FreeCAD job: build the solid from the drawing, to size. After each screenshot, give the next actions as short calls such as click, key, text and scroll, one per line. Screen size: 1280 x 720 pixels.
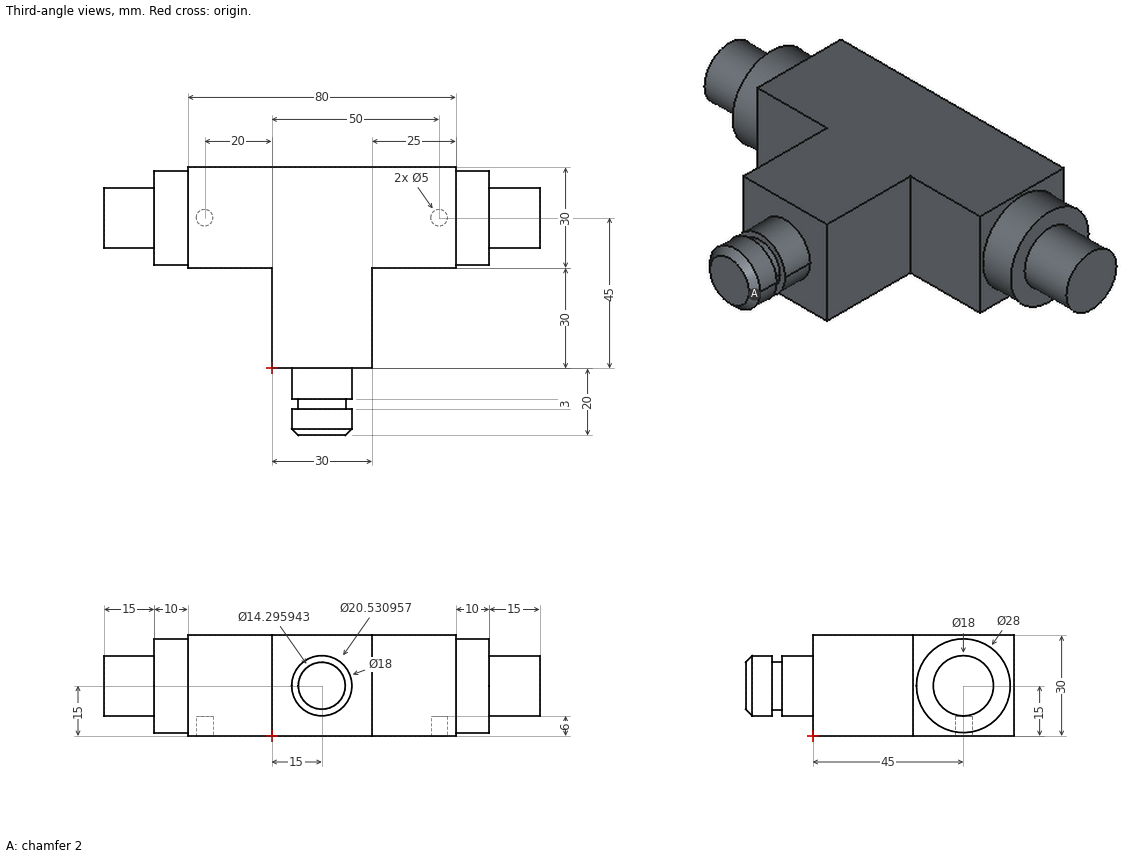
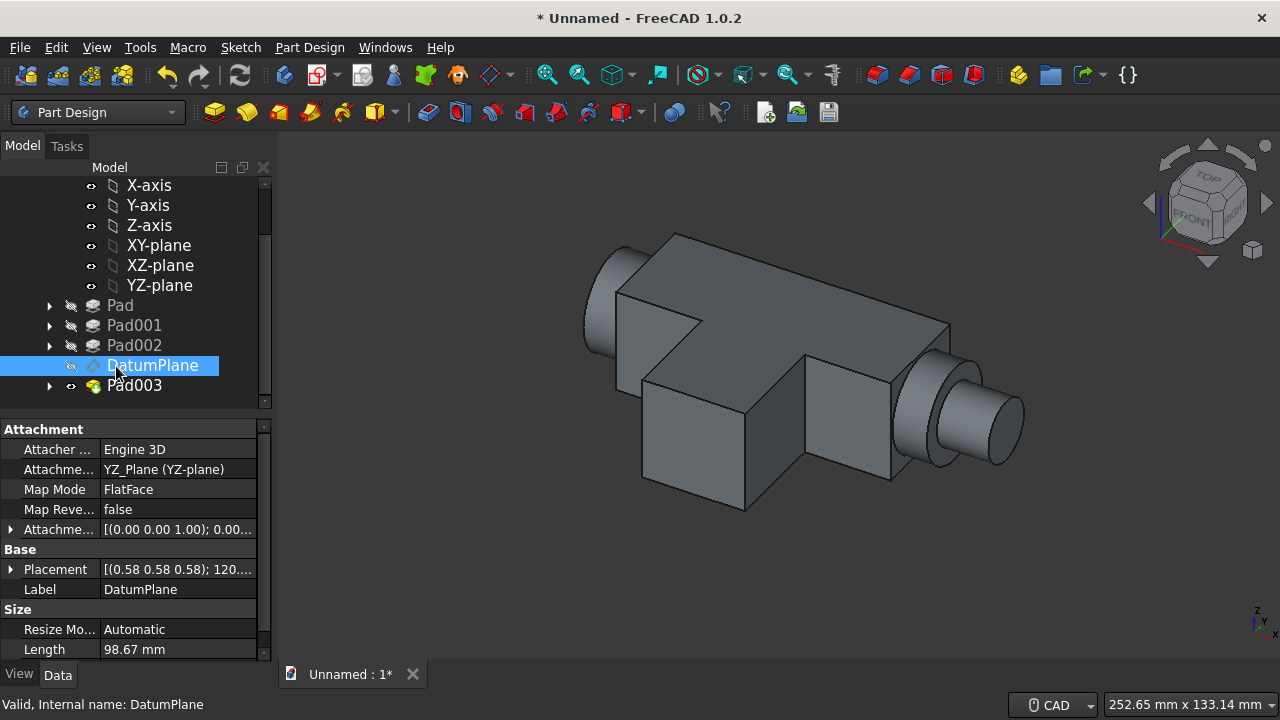
scroll(160, 281, down, 3)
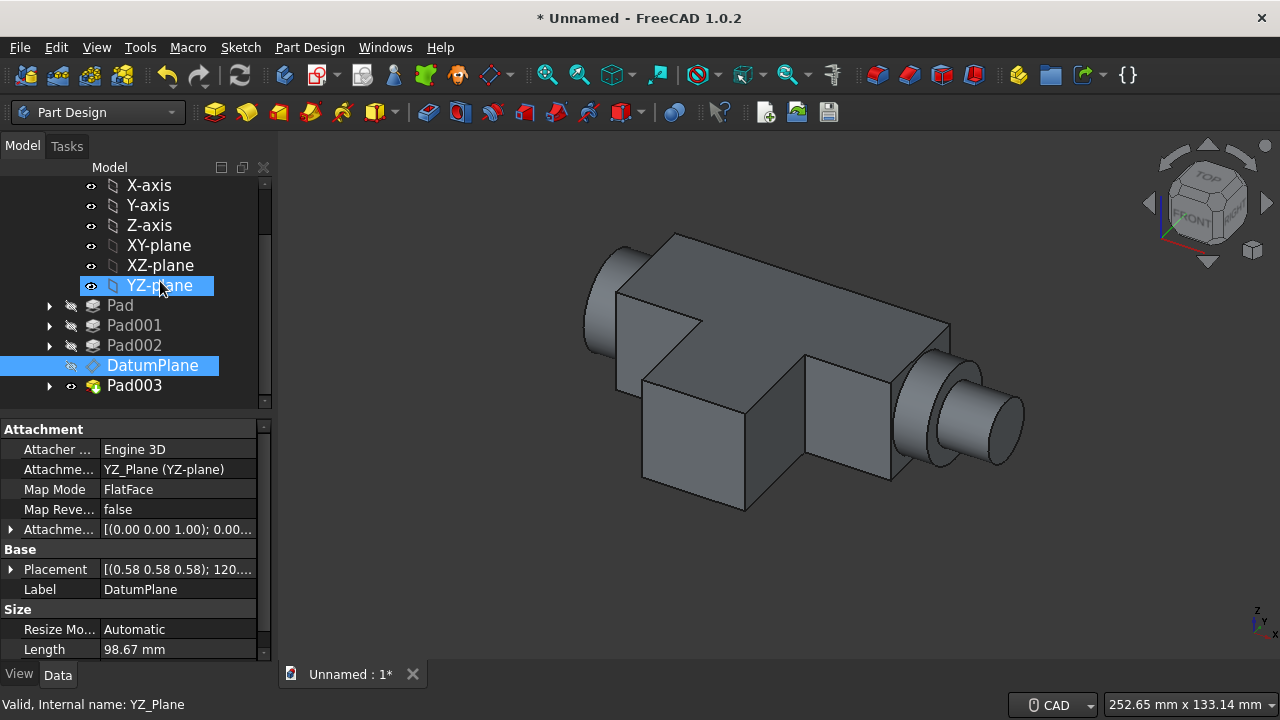
scroll(160, 281, up, 15)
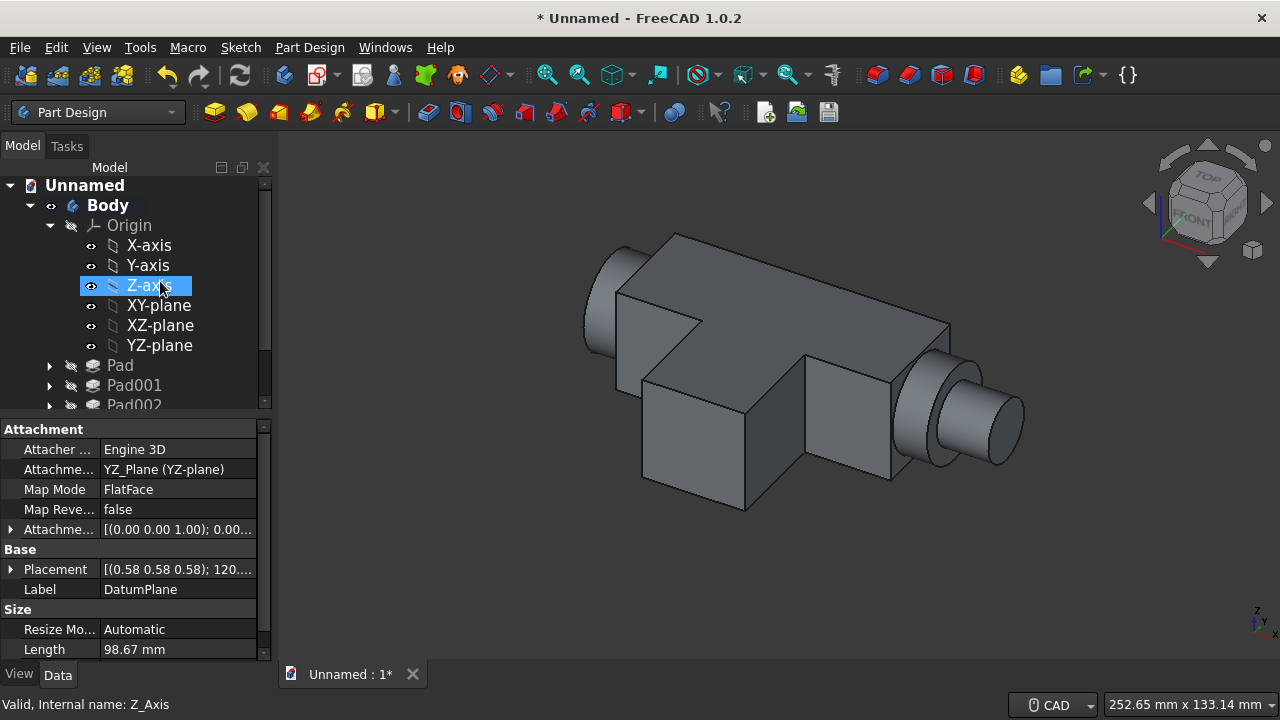
click(136, 346)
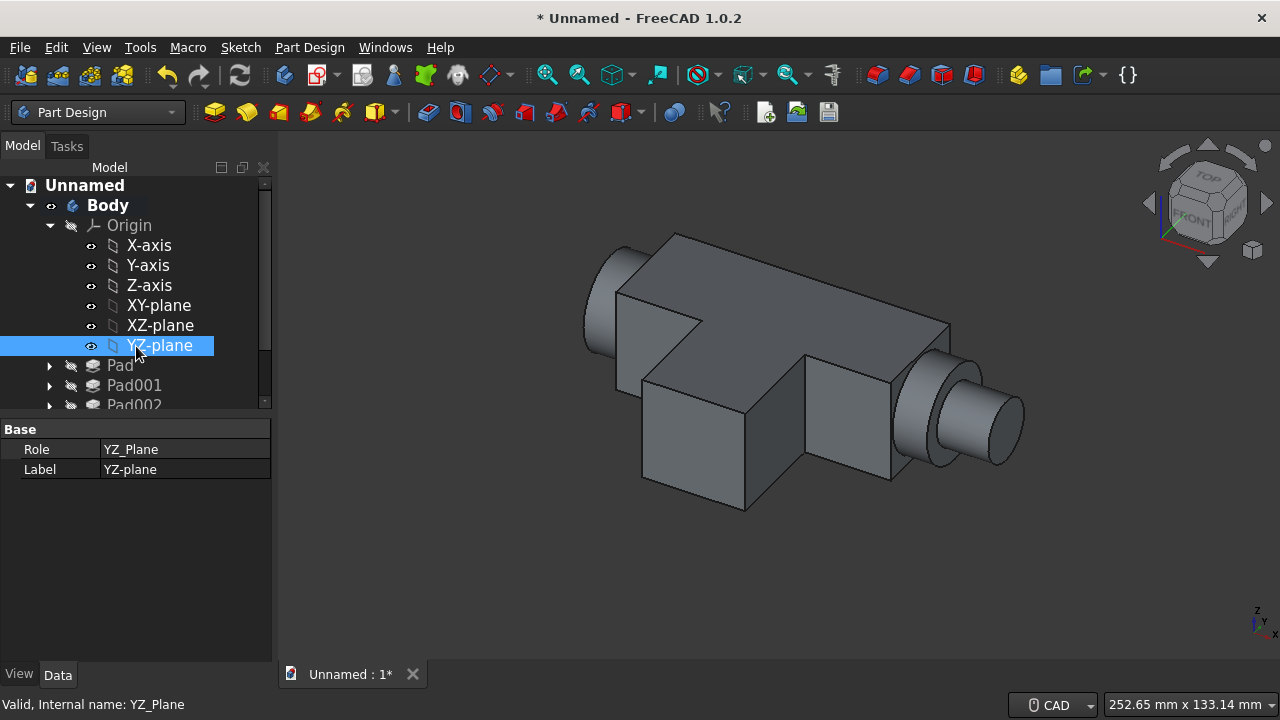
click(490, 76)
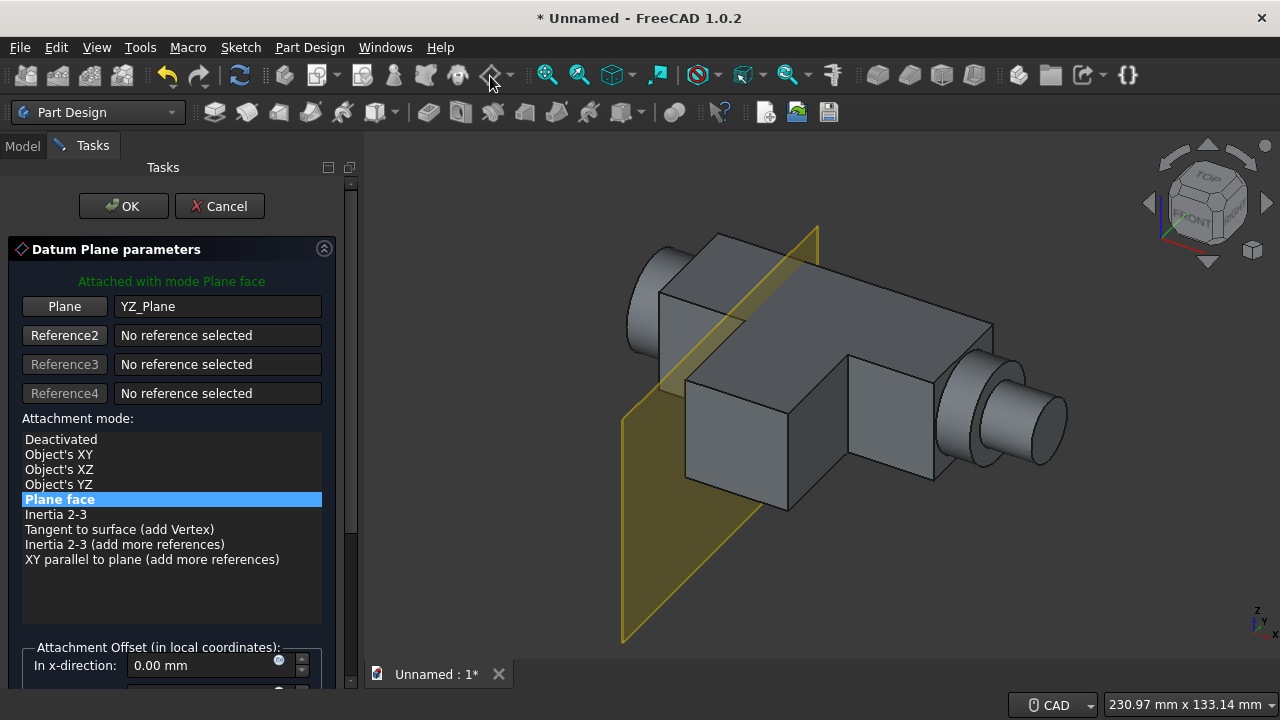
scroll(351, 432, down, 2)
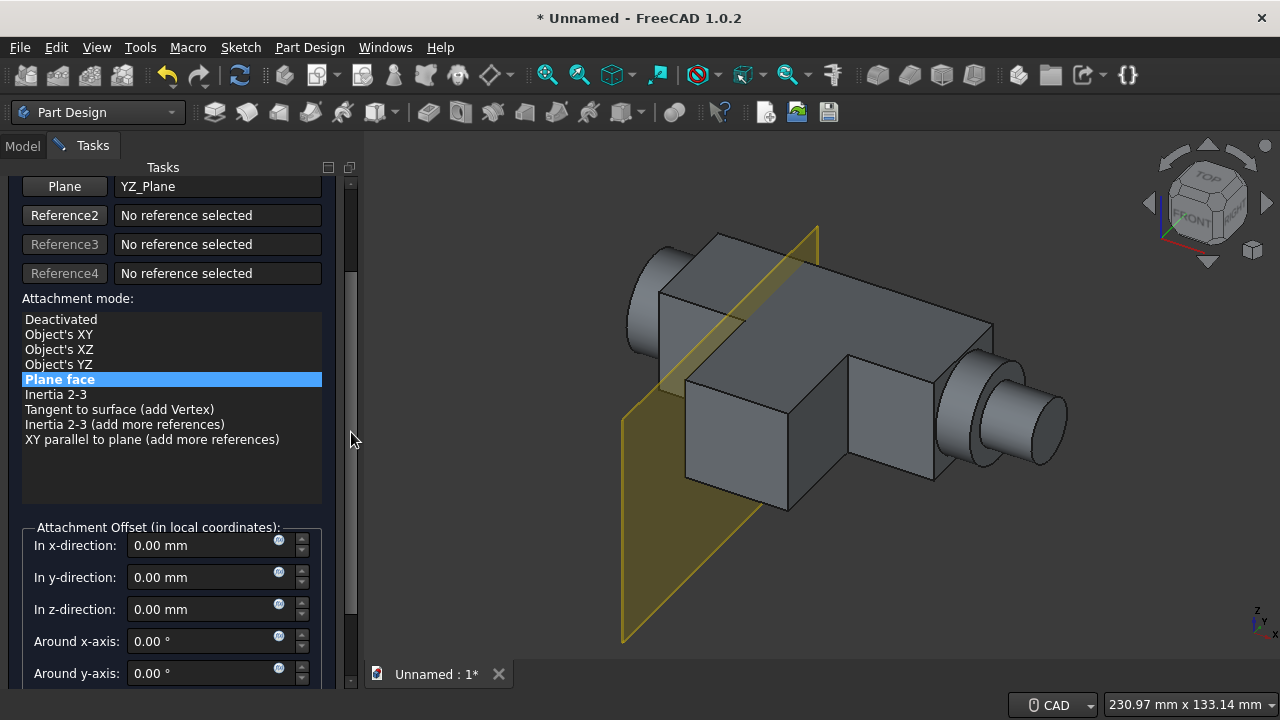
triple_click(210, 609)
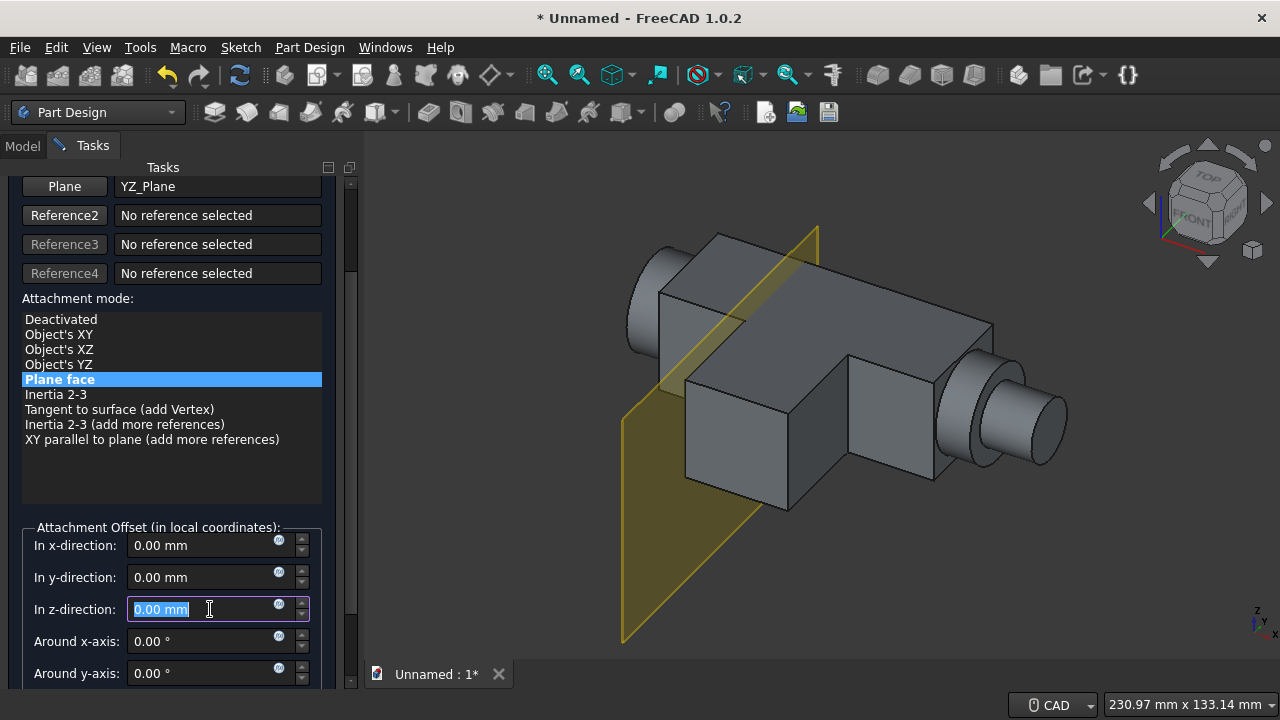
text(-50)
key(Tab)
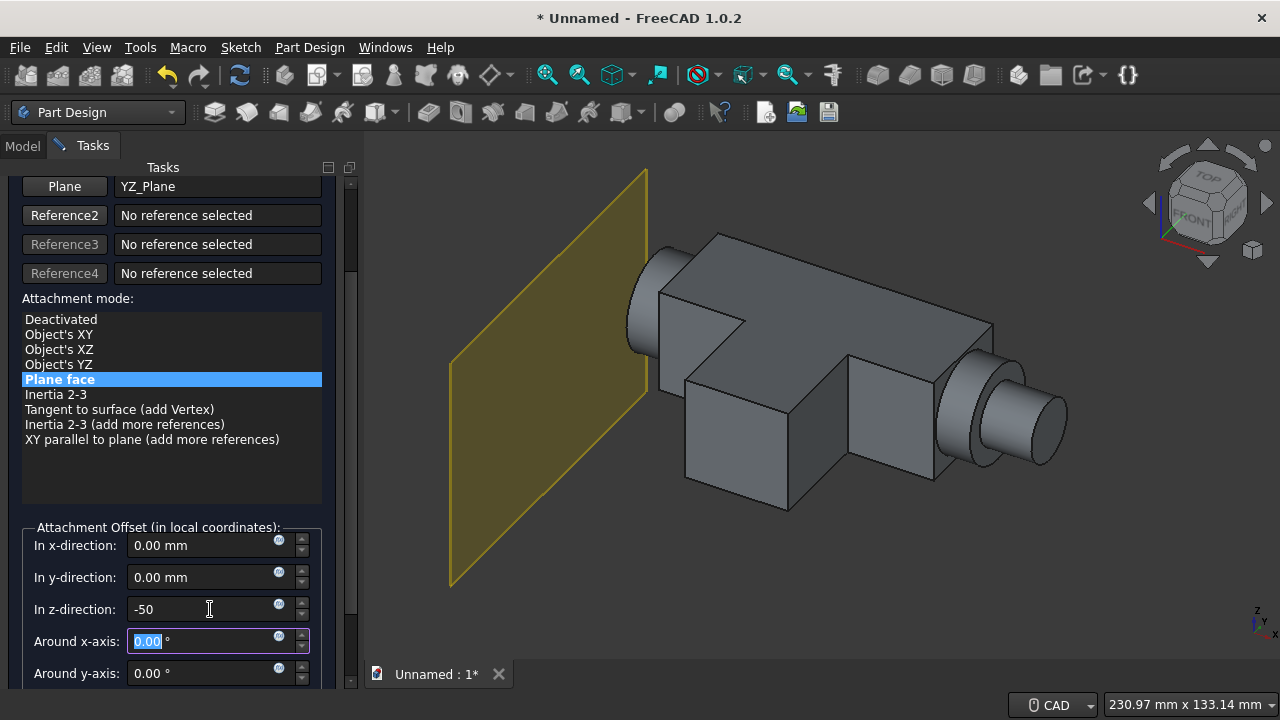
scroll(351, 432, up, 3)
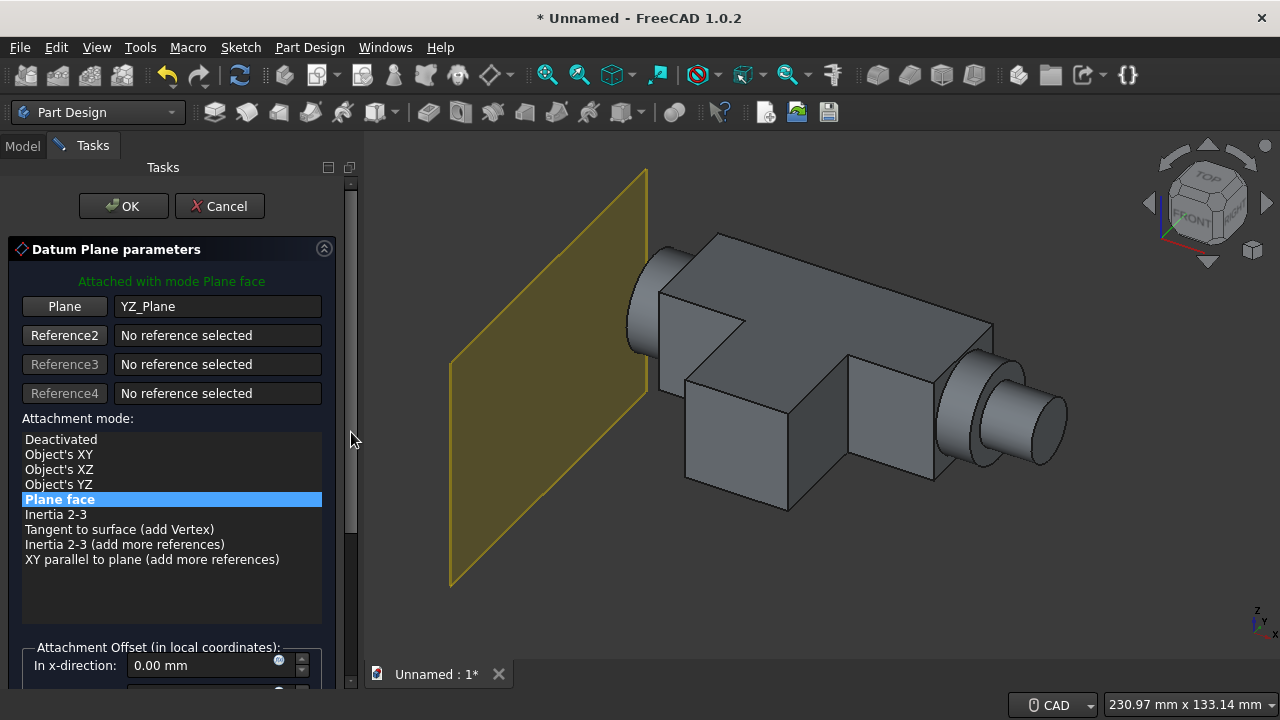
click(124, 206)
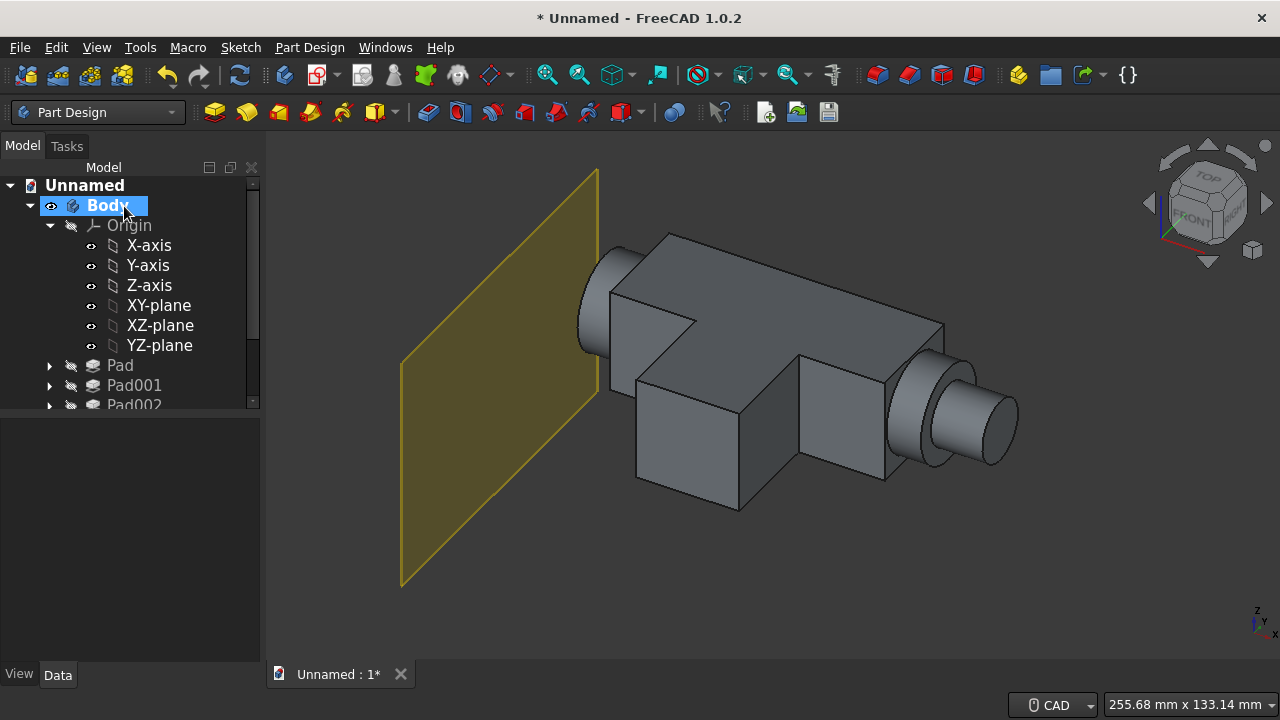
scroll(100, 301, down, 3)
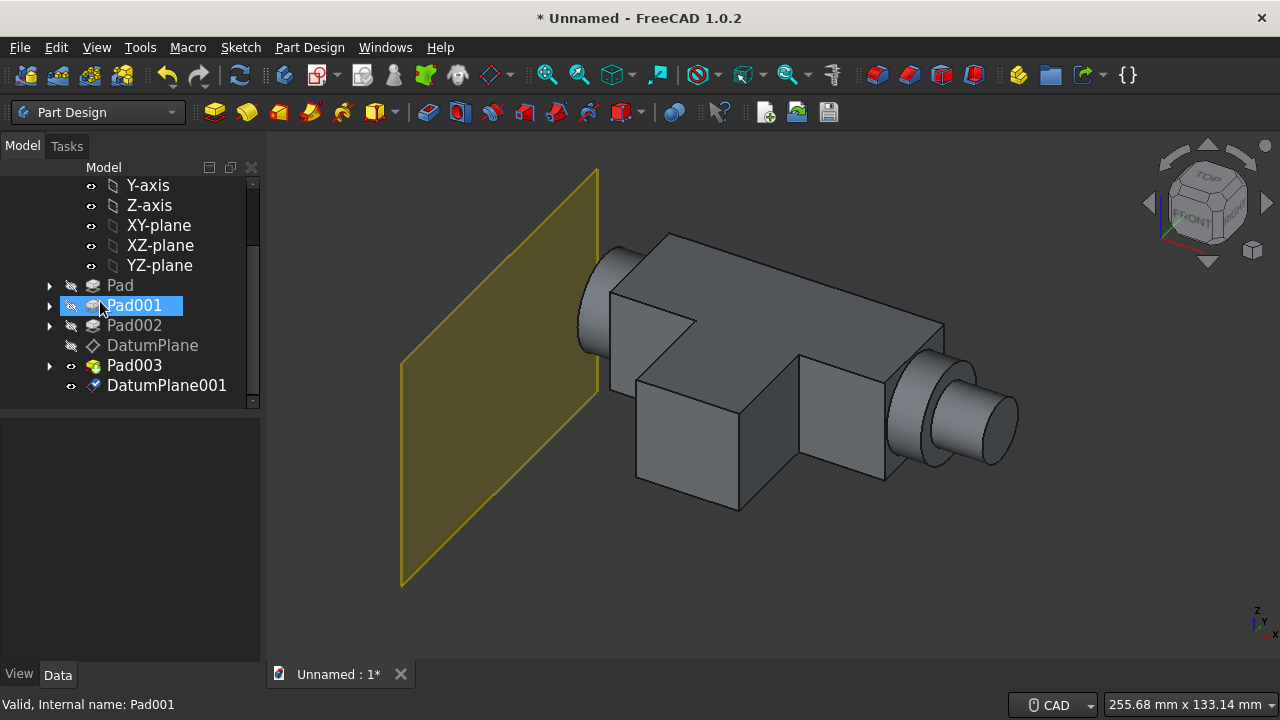
click(116, 386)